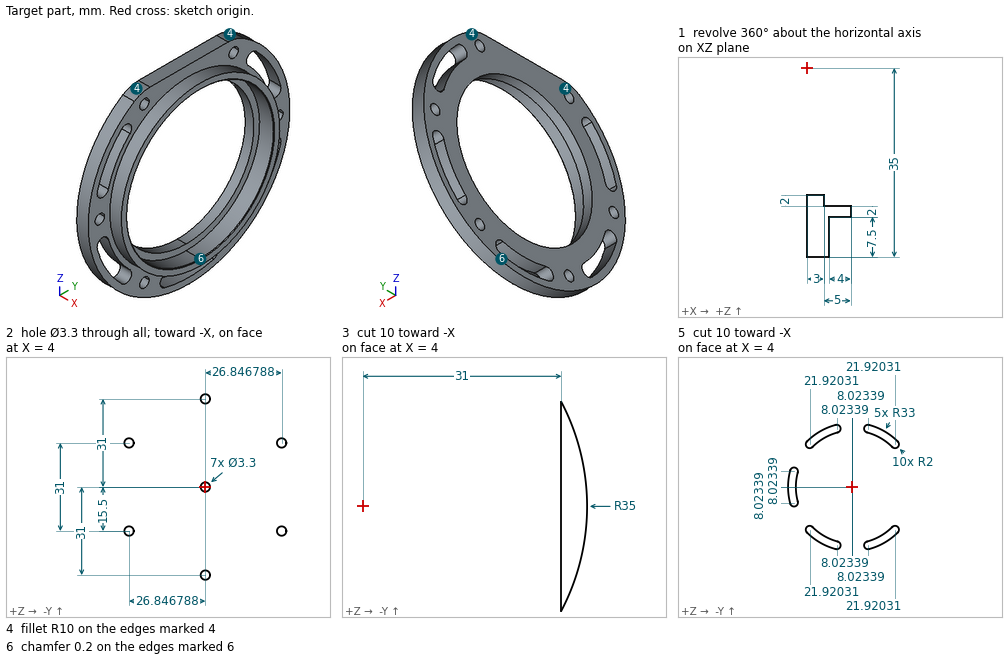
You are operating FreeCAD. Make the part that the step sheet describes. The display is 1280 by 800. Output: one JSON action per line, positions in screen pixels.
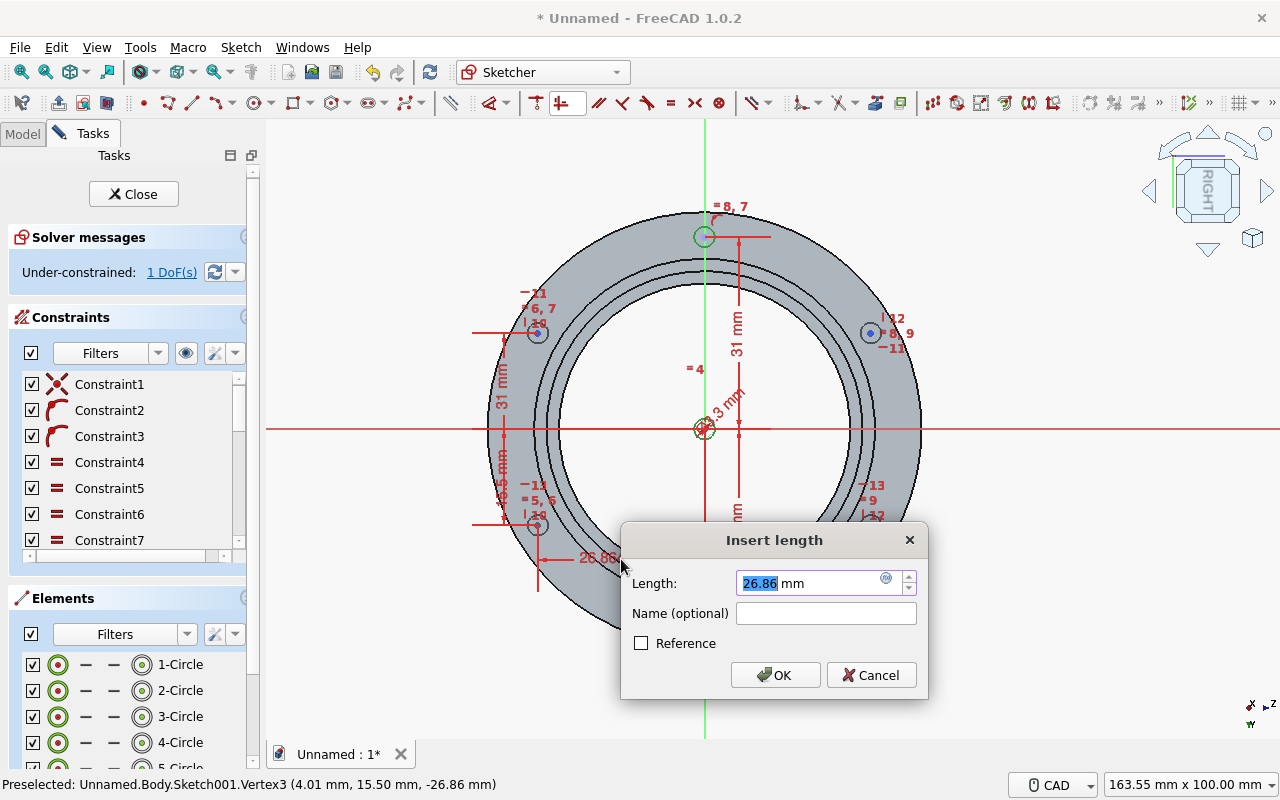
{"action": "type", "text": "26.846788"}
{"action": "key", "text": "Return"}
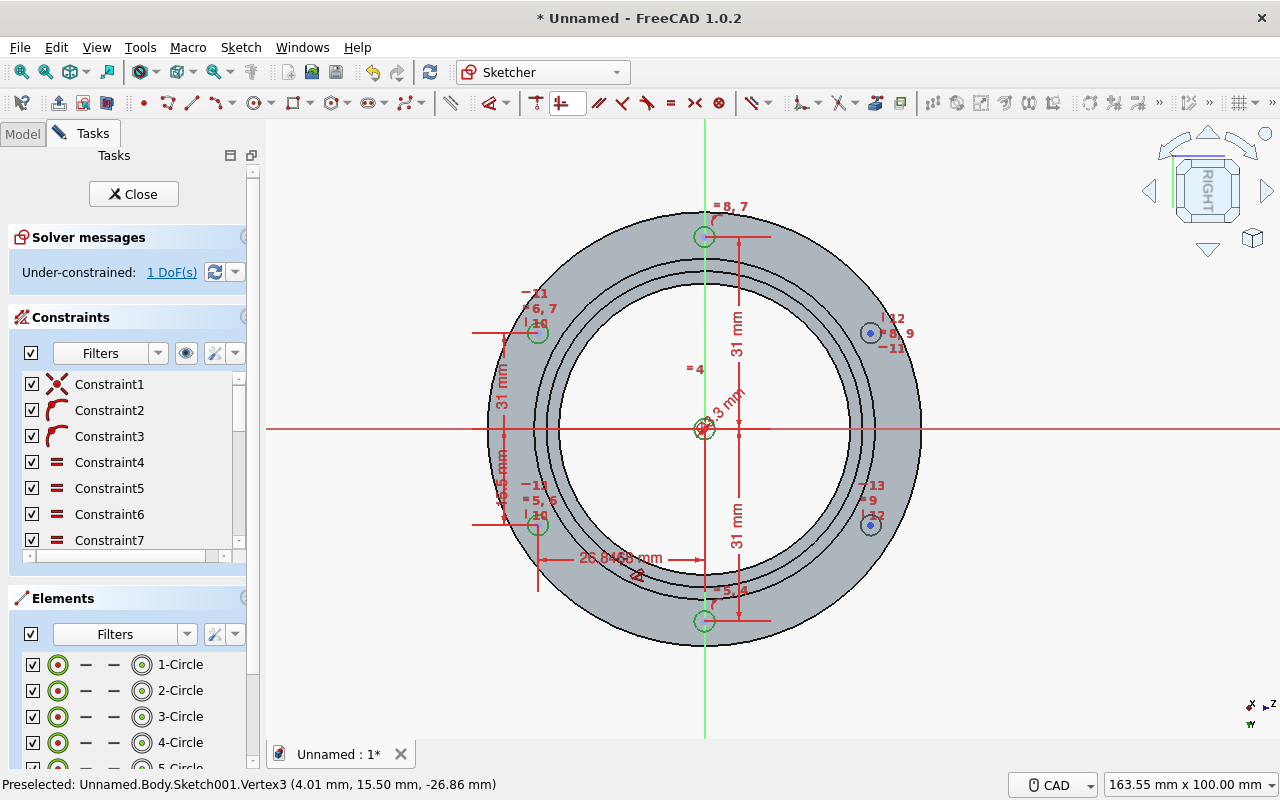
{"action": "left_click", "coordinate": [871, 333]}
{"action": "left_click", "coordinate": [788, 299]}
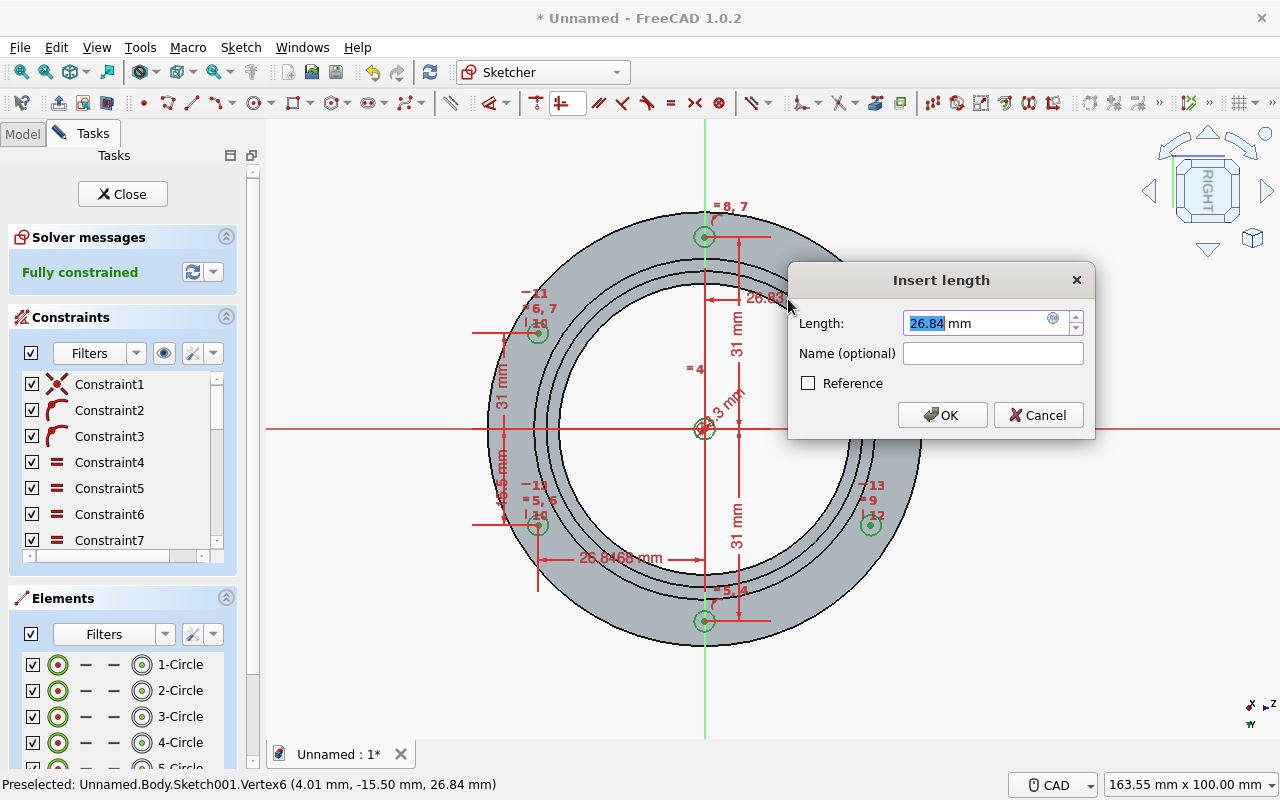
{"action": "type", "text": "26.846788"}
{"action": "key", "text": "Return"}
{"action": "key", "text": "Escape"}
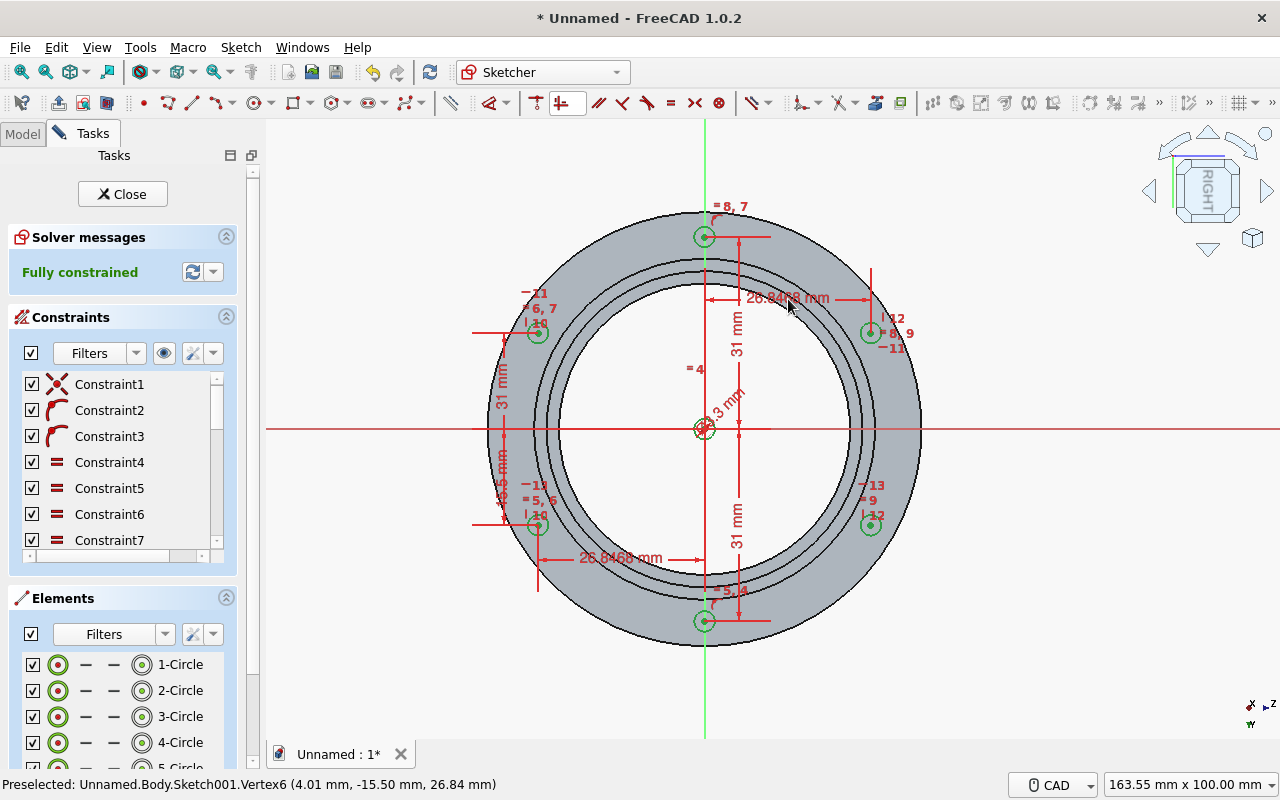
{"action": "left_click", "coordinate": [123, 194]}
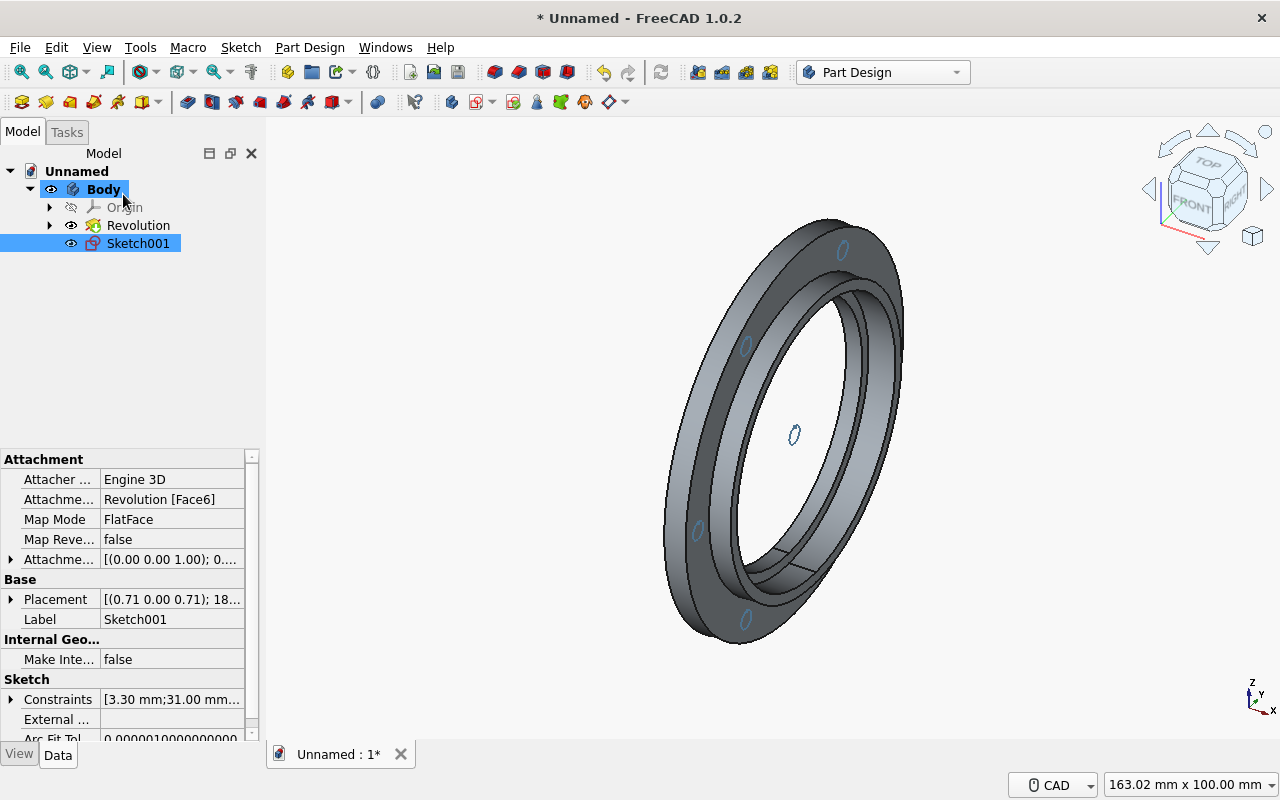
{"action": "left_click", "coordinate": [212, 102]}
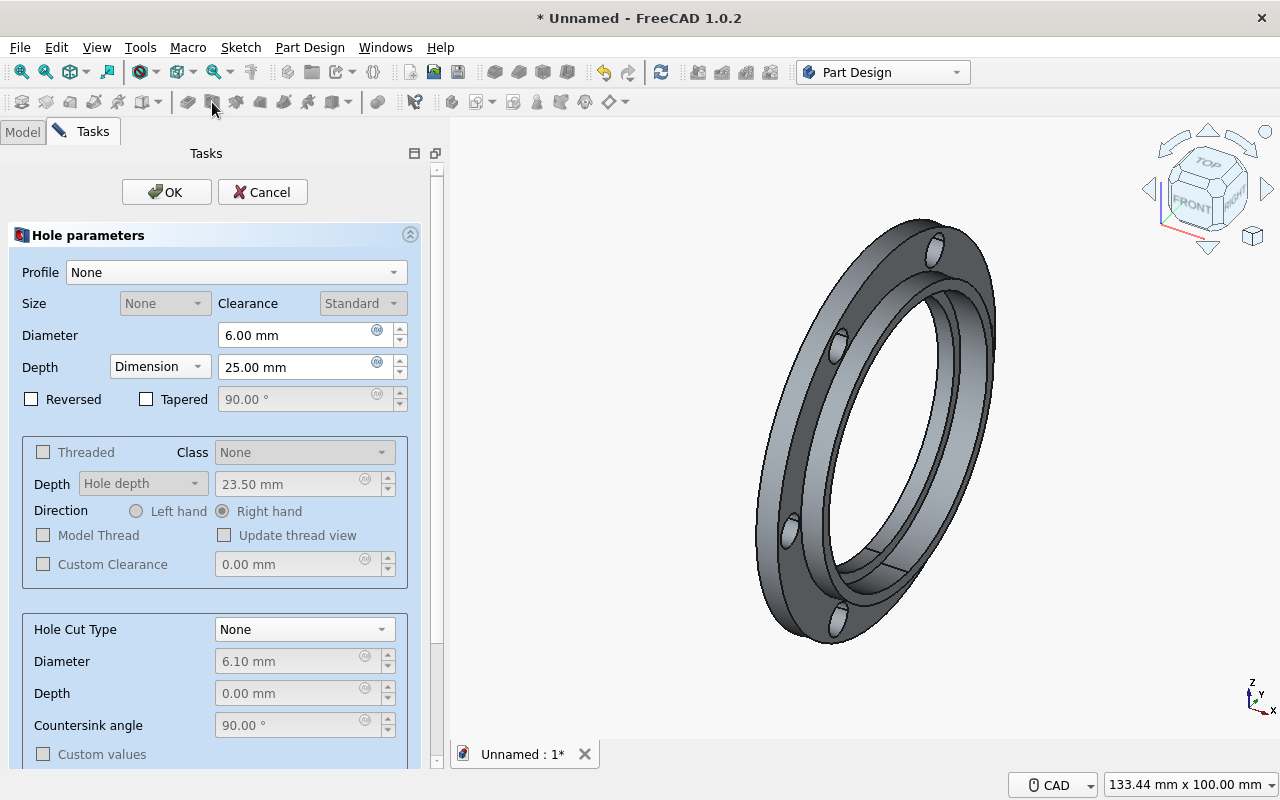
{"action": "triple_click", "coordinate": [305, 335]}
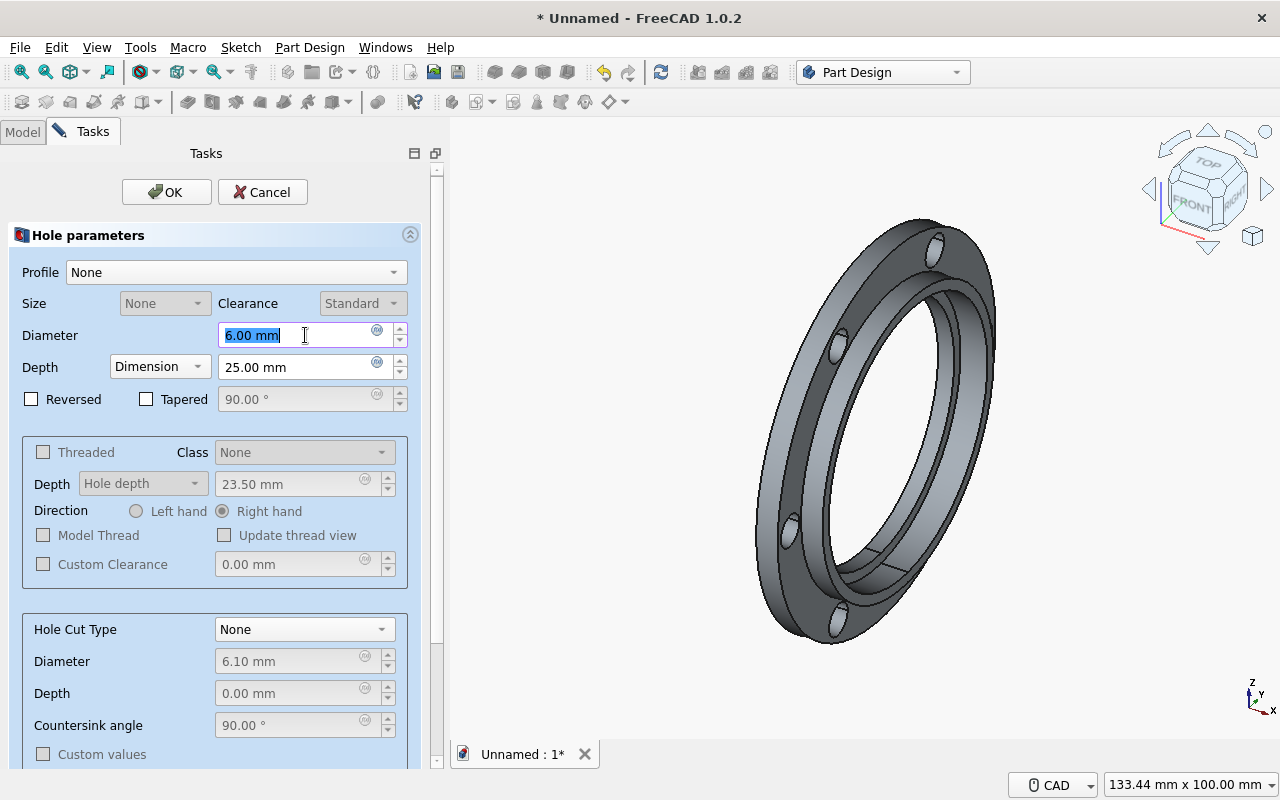
{"action": "type", "text": "3.3"}
{"action": "key", "text": "Tab"}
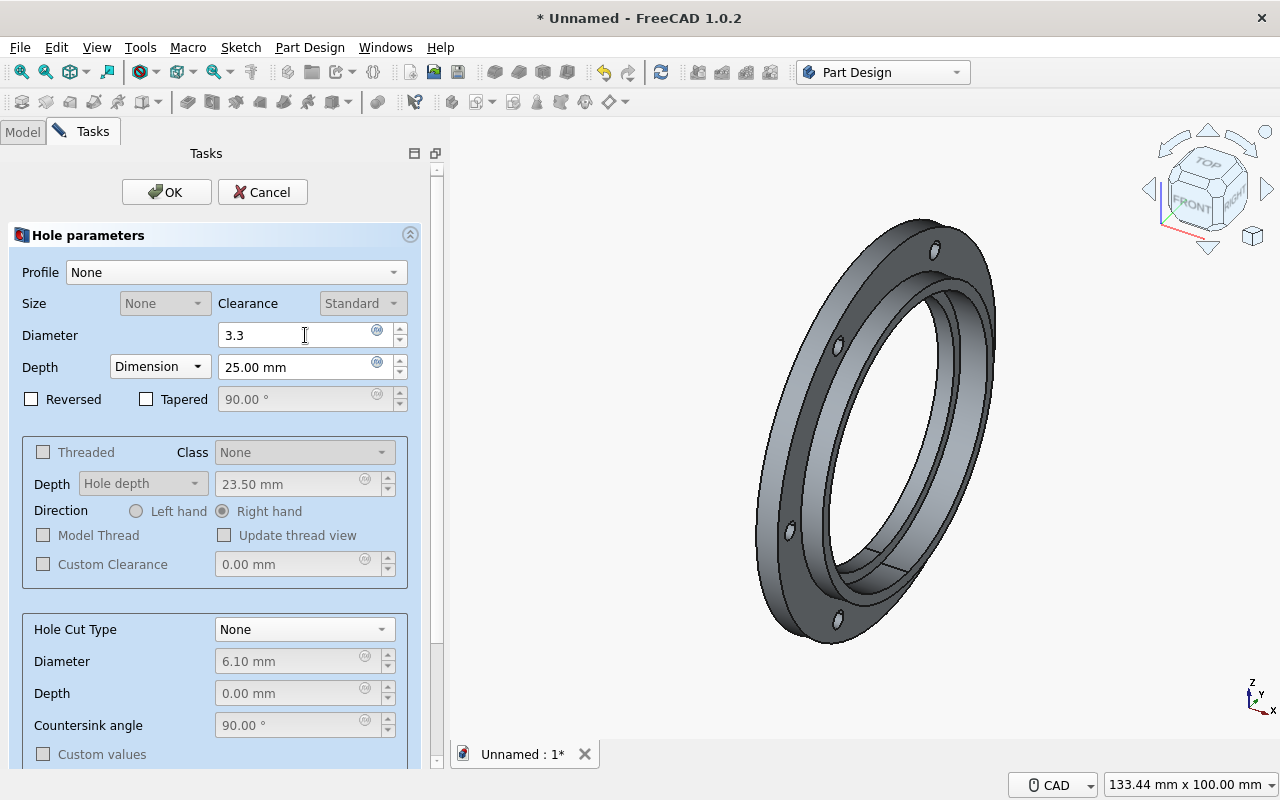
{"action": "left_click", "coordinate": [161, 366]}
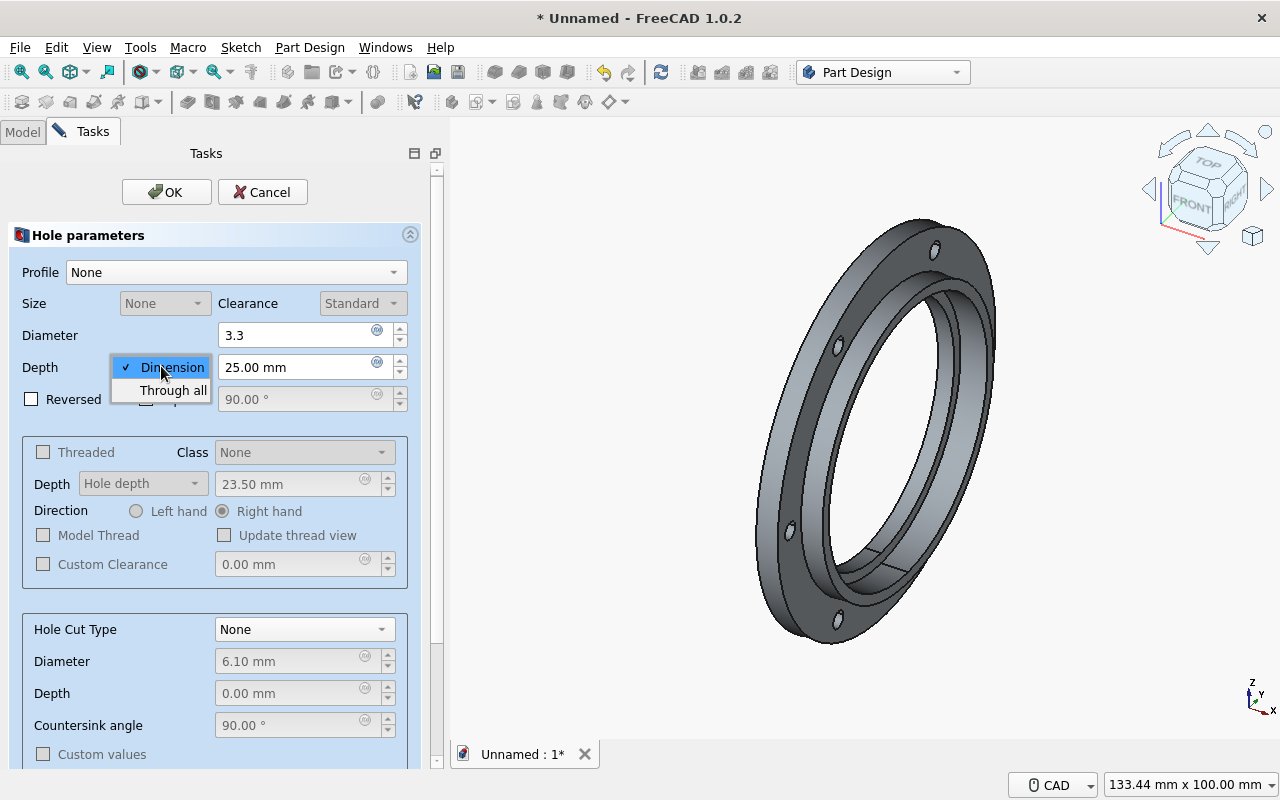
{"action": "left_click", "coordinate": [160, 390]}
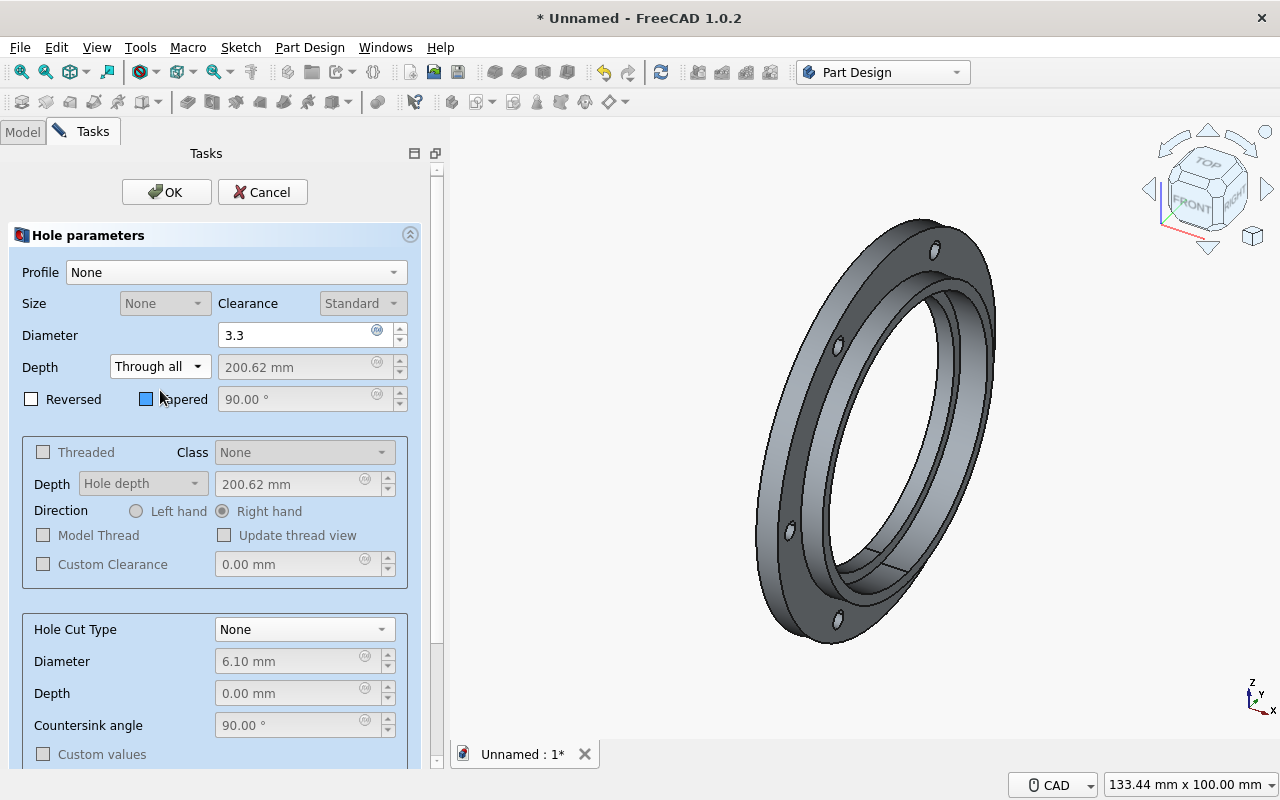
{"action": "left_click", "coordinate": [167, 192]}